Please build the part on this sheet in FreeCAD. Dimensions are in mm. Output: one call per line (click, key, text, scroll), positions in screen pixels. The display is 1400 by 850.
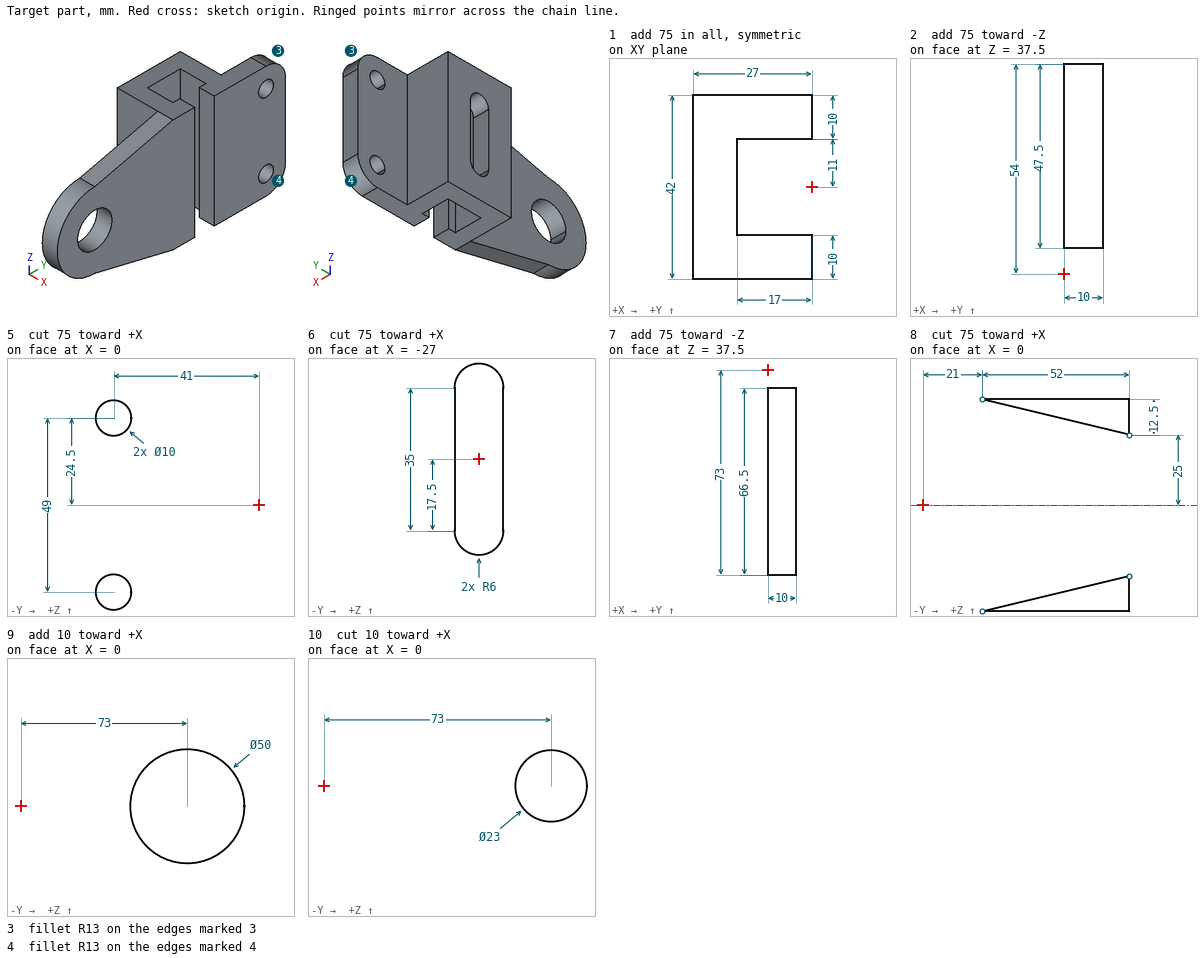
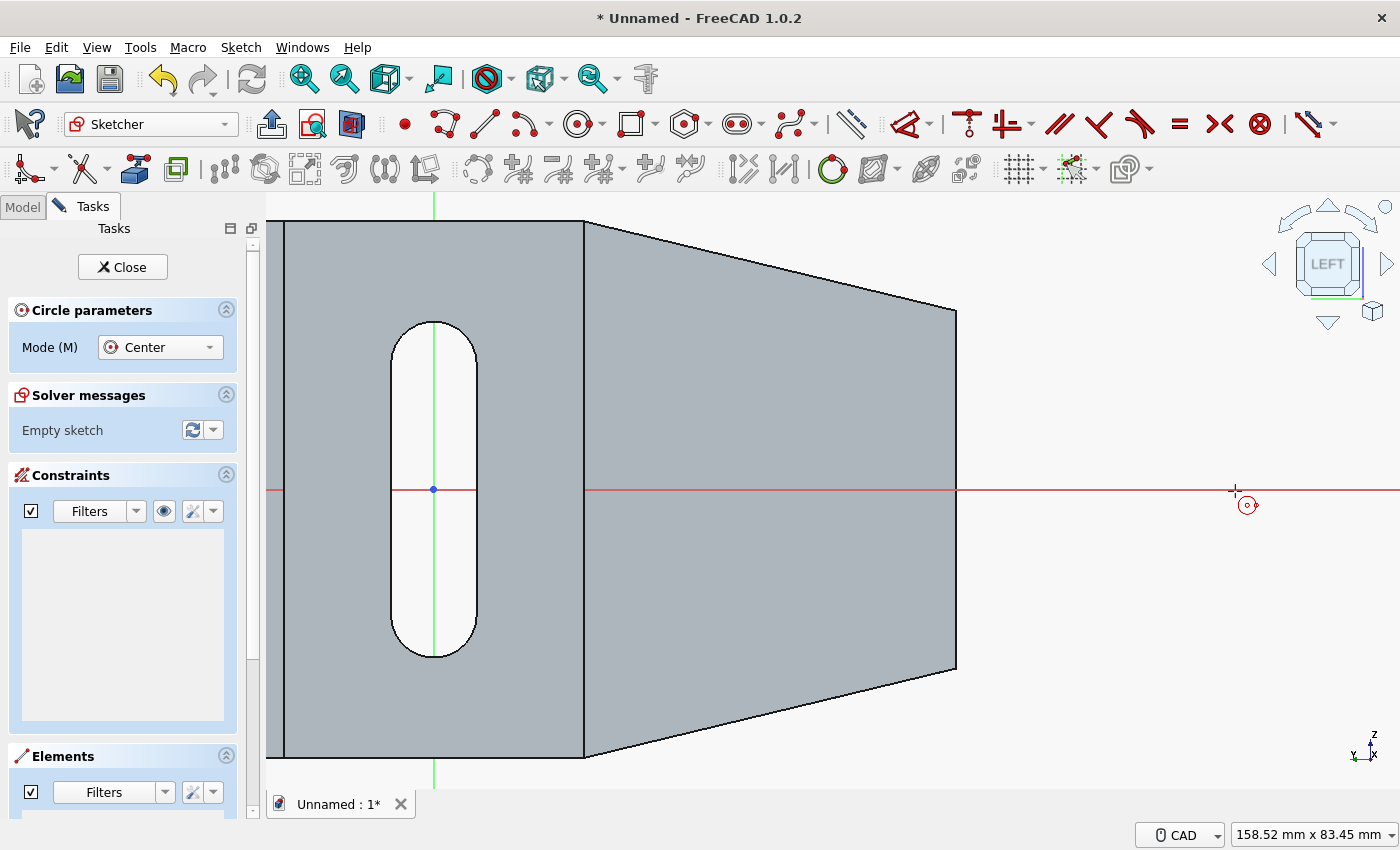
click(956, 490)
click(1083, 363)
key(Escape)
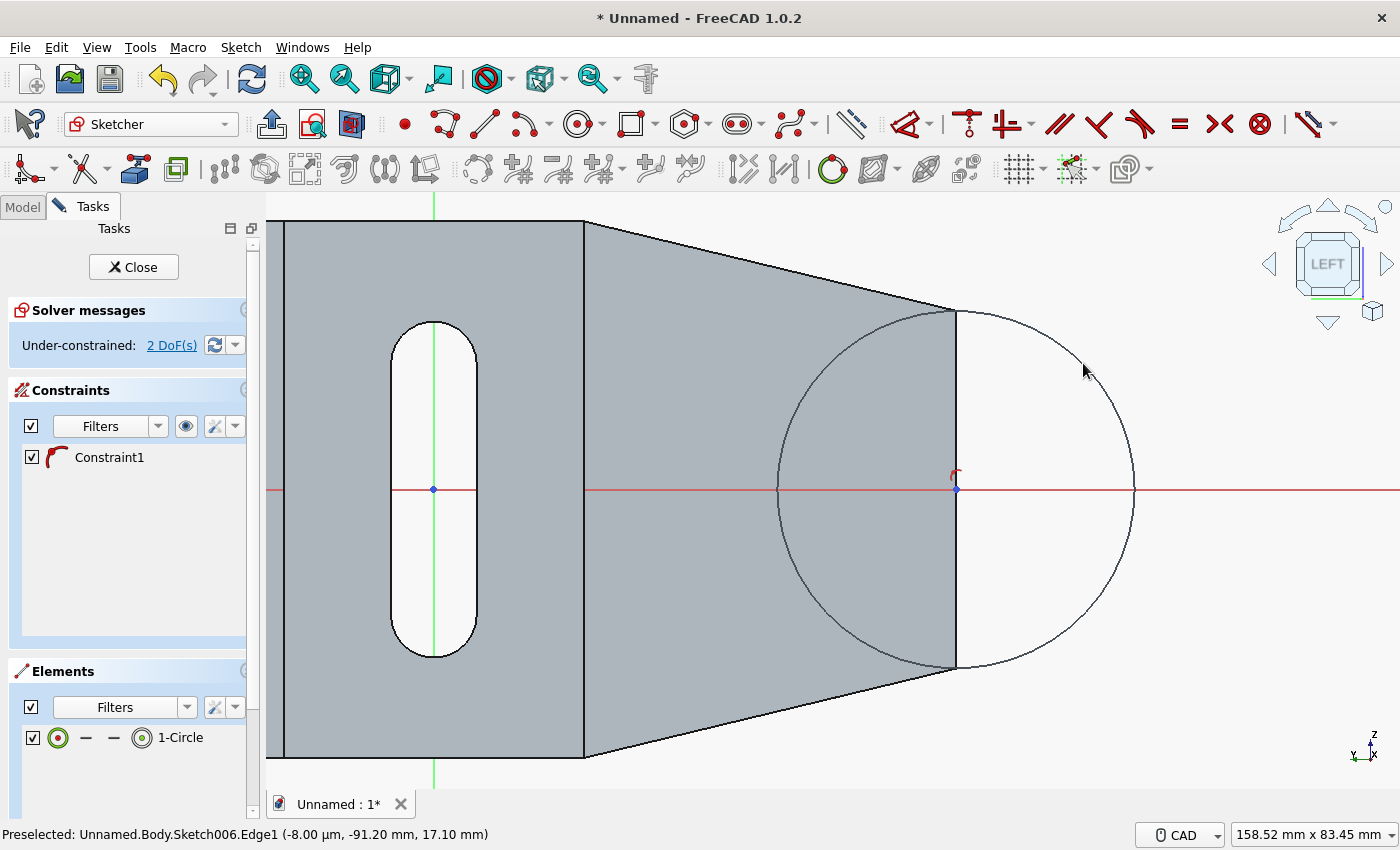
click(906, 124)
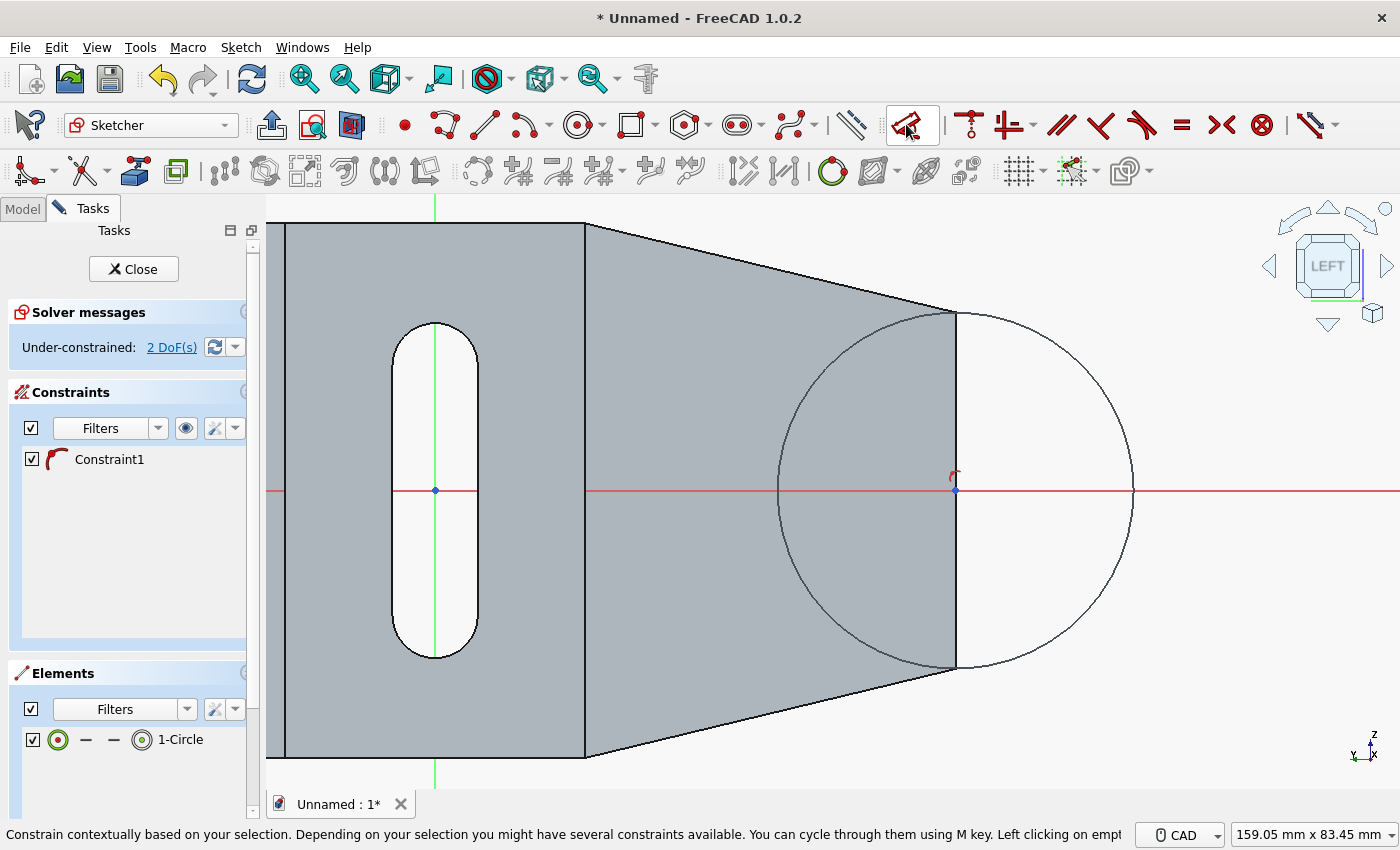
click(1081, 364)
click(1104, 341)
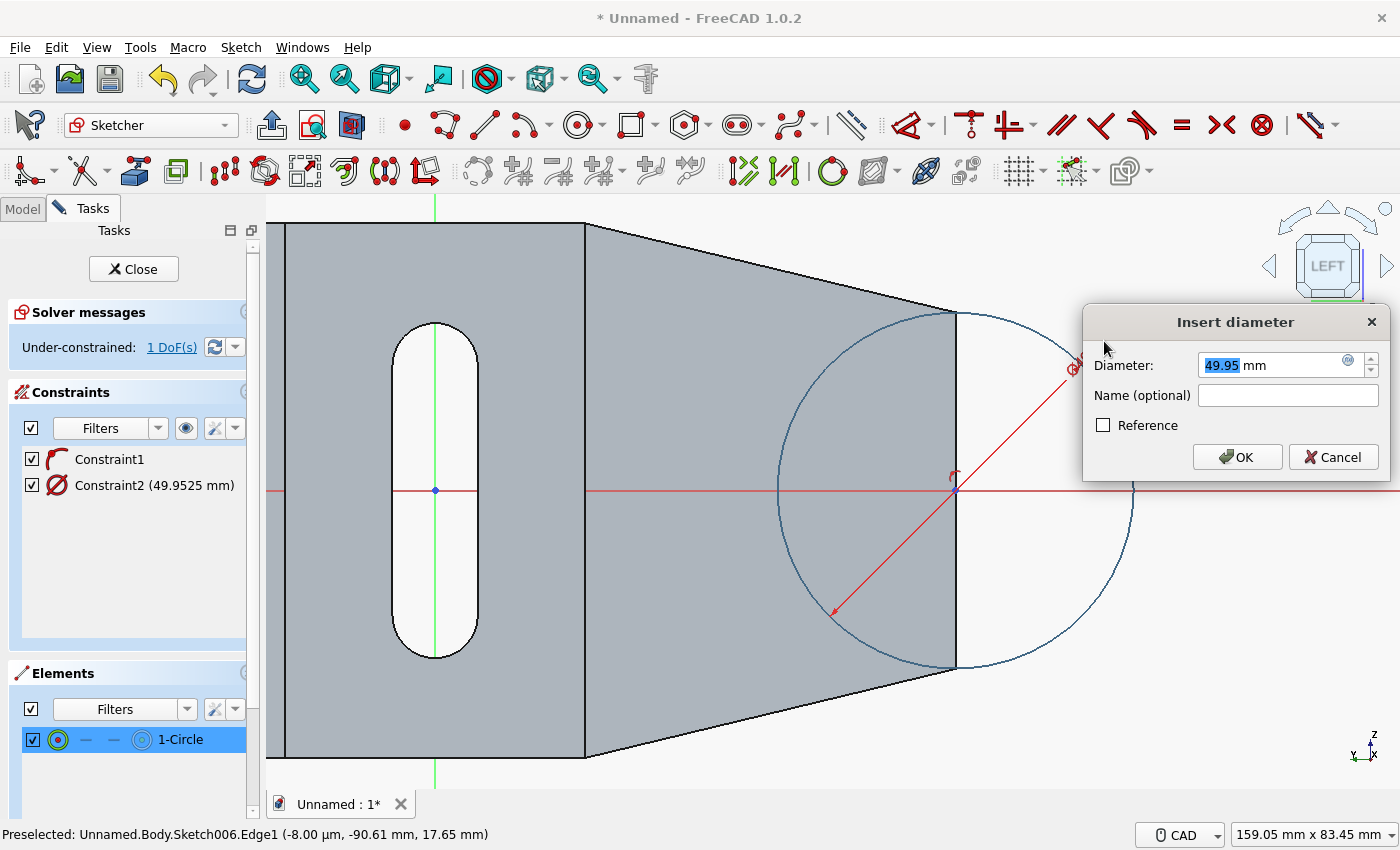
text(50)
key(Return)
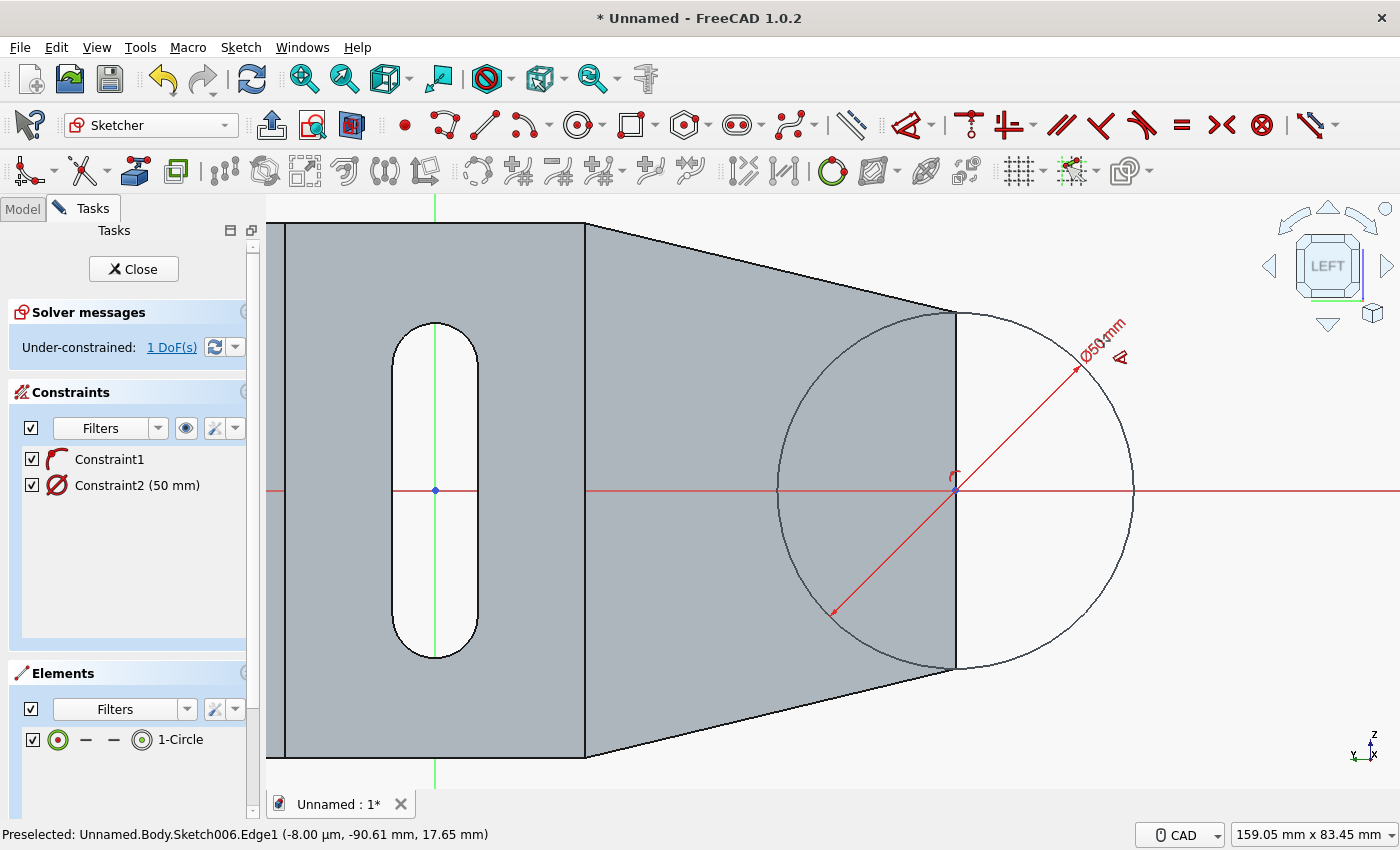
click(956, 491)
click(695, 525)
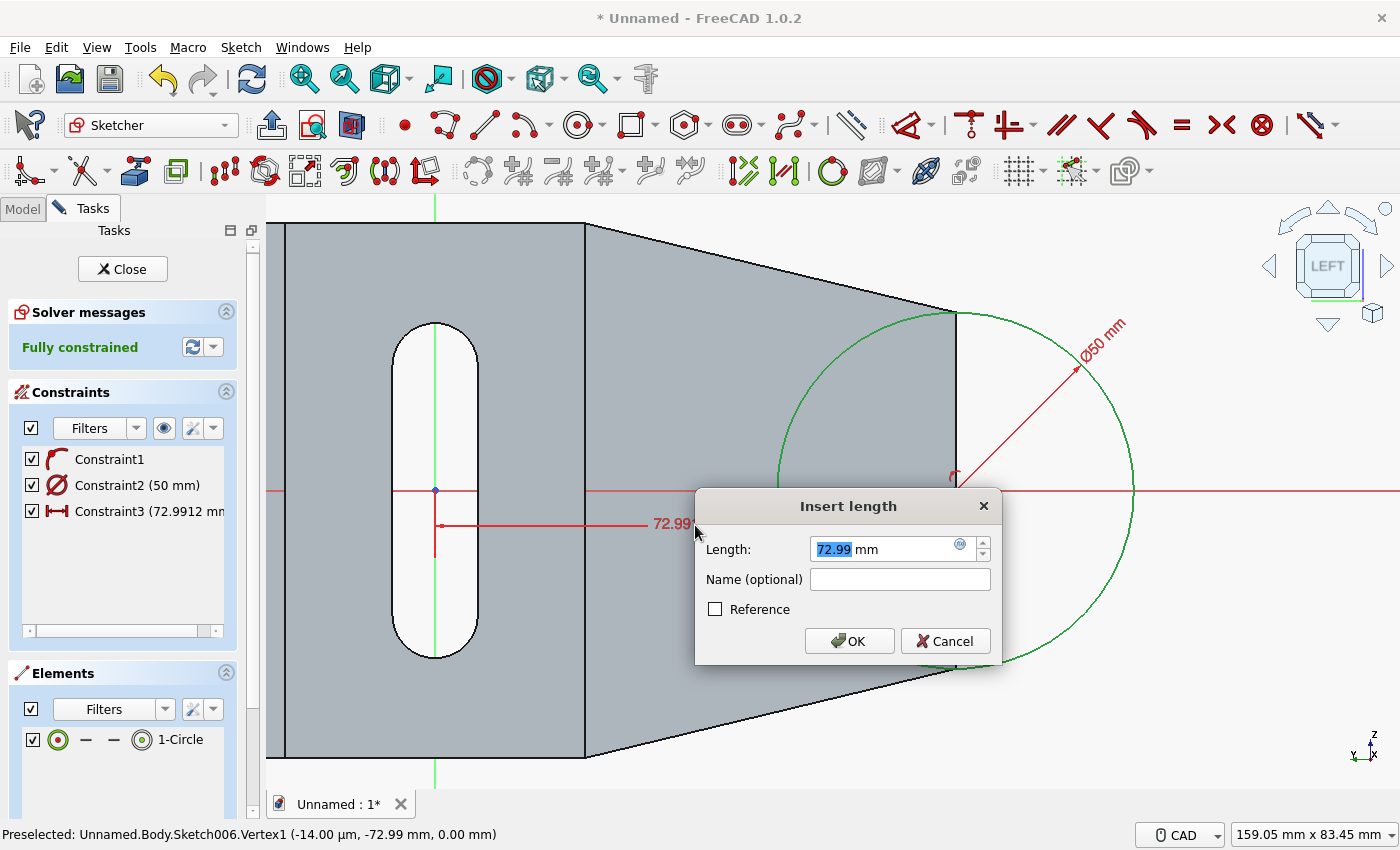
text(73)
key(Return)
key(Escape)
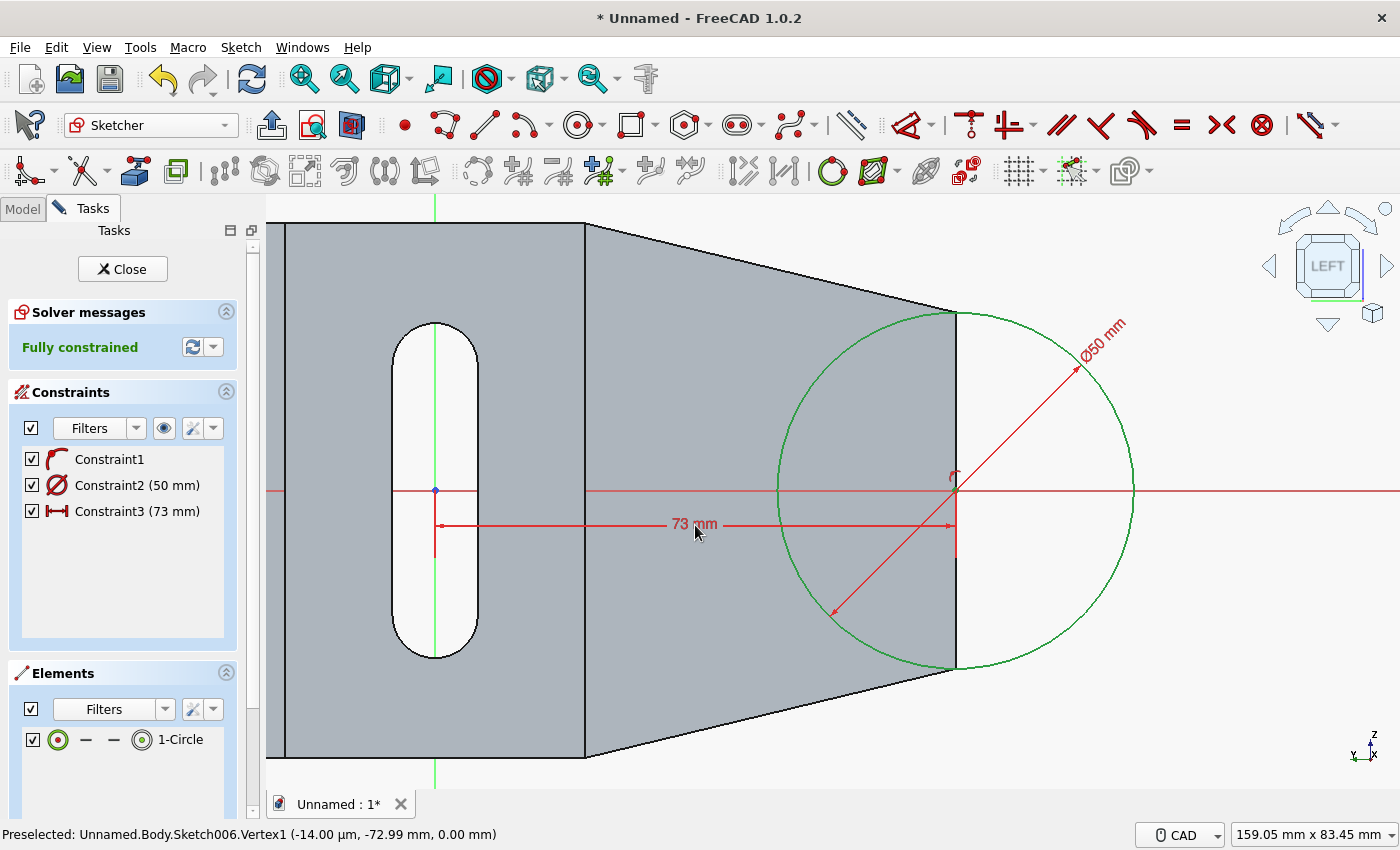
click(123, 269)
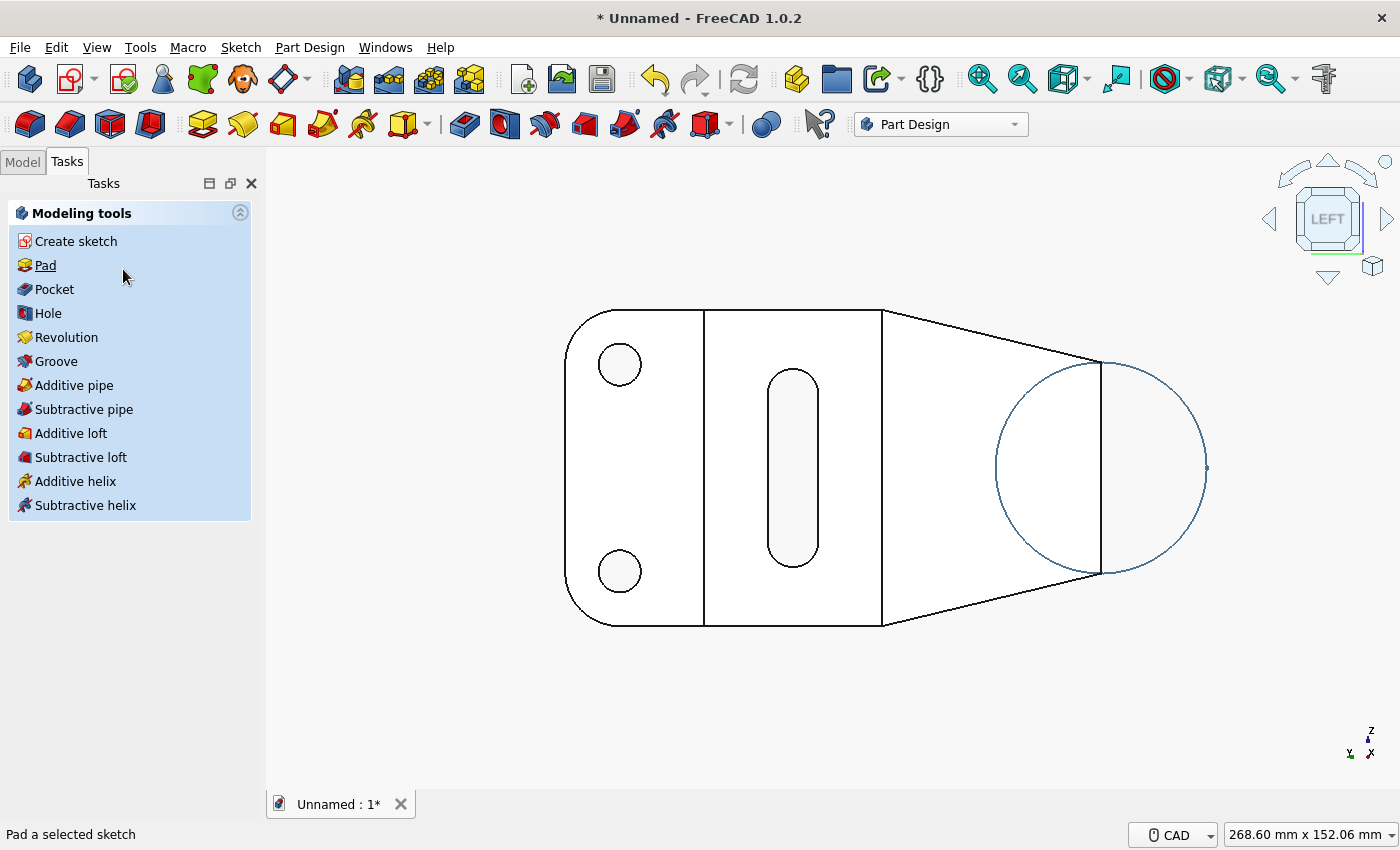
click(204, 124)